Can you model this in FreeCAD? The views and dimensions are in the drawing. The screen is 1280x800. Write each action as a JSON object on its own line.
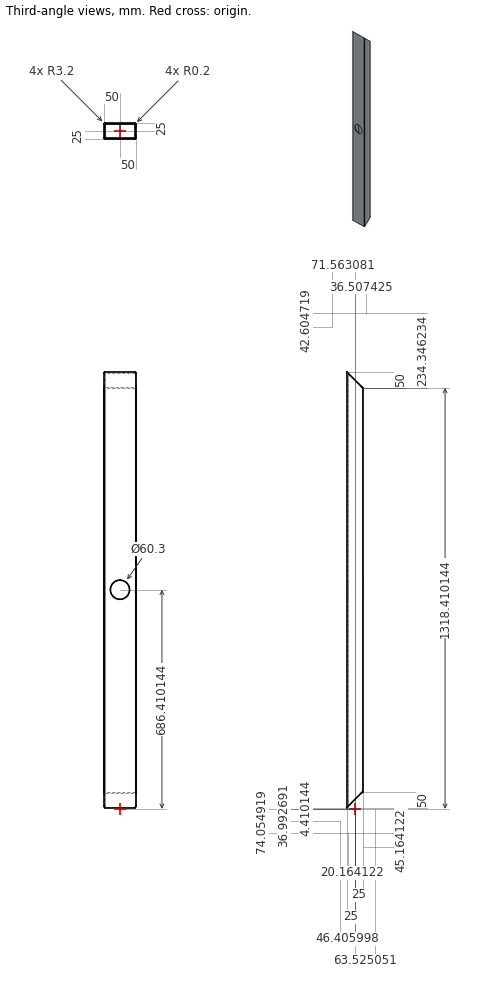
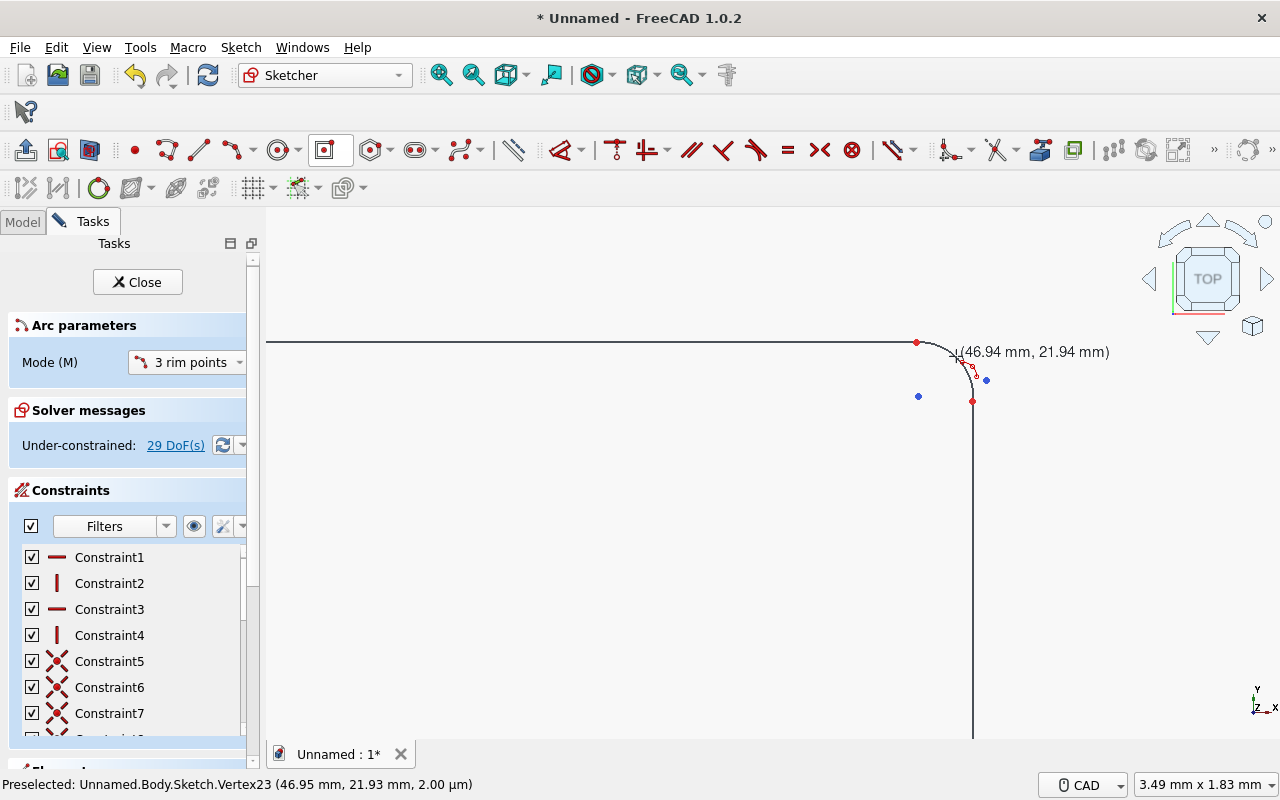
{"action": "scroll", "coordinate": [704, 473], "scroll_direction": "down", "scroll_amount": 15}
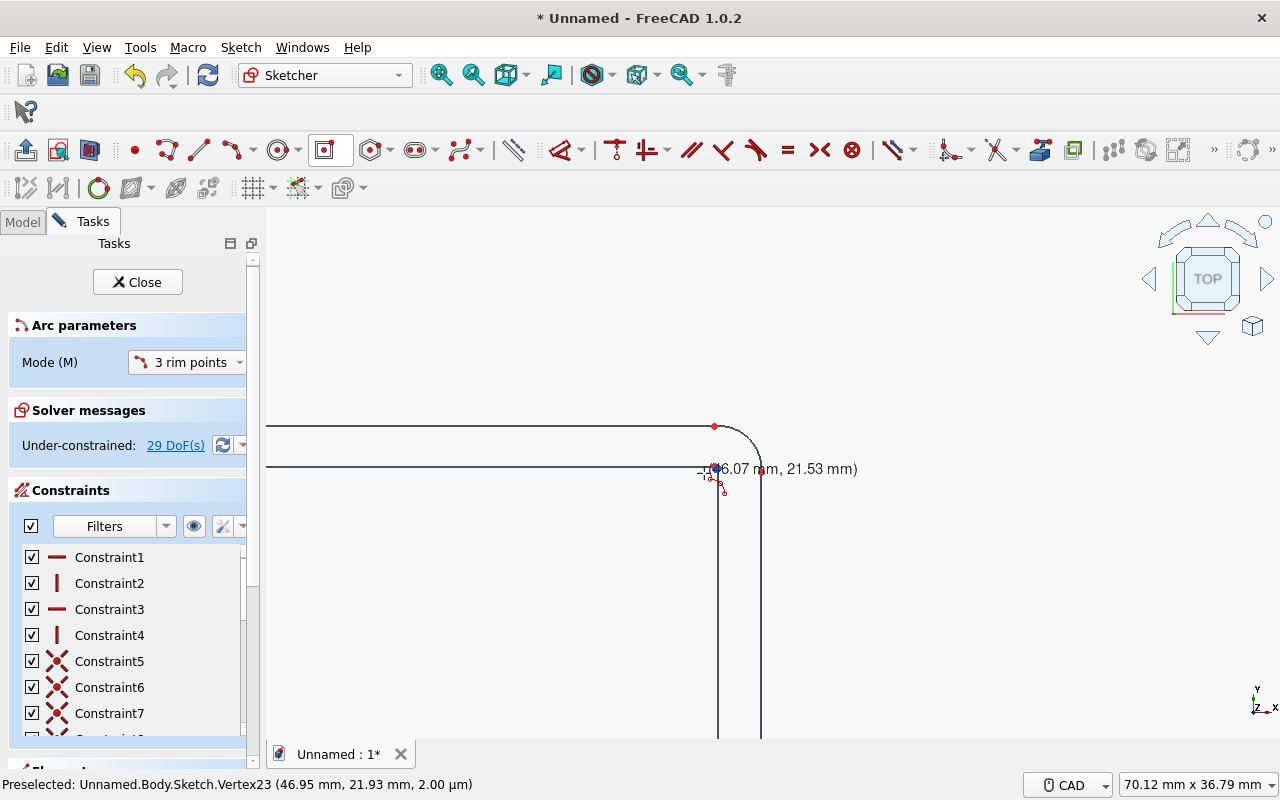
{"action": "scroll", "coordinate": [1092, 291], "scroll_direction": "down", "scroll_amount": 5}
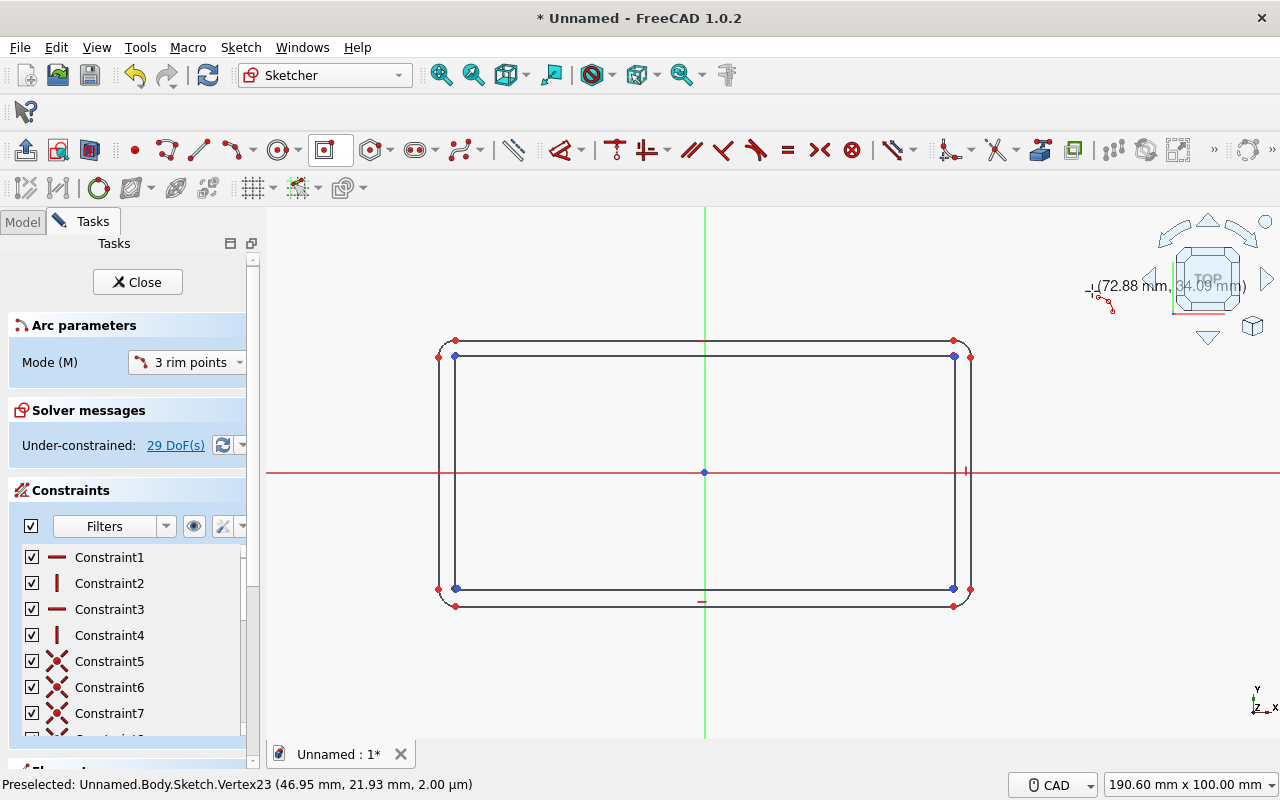
{"action": "scroll", "coordinate": [955, 589], "scroll_direction": "up", "scroll_amount": 14}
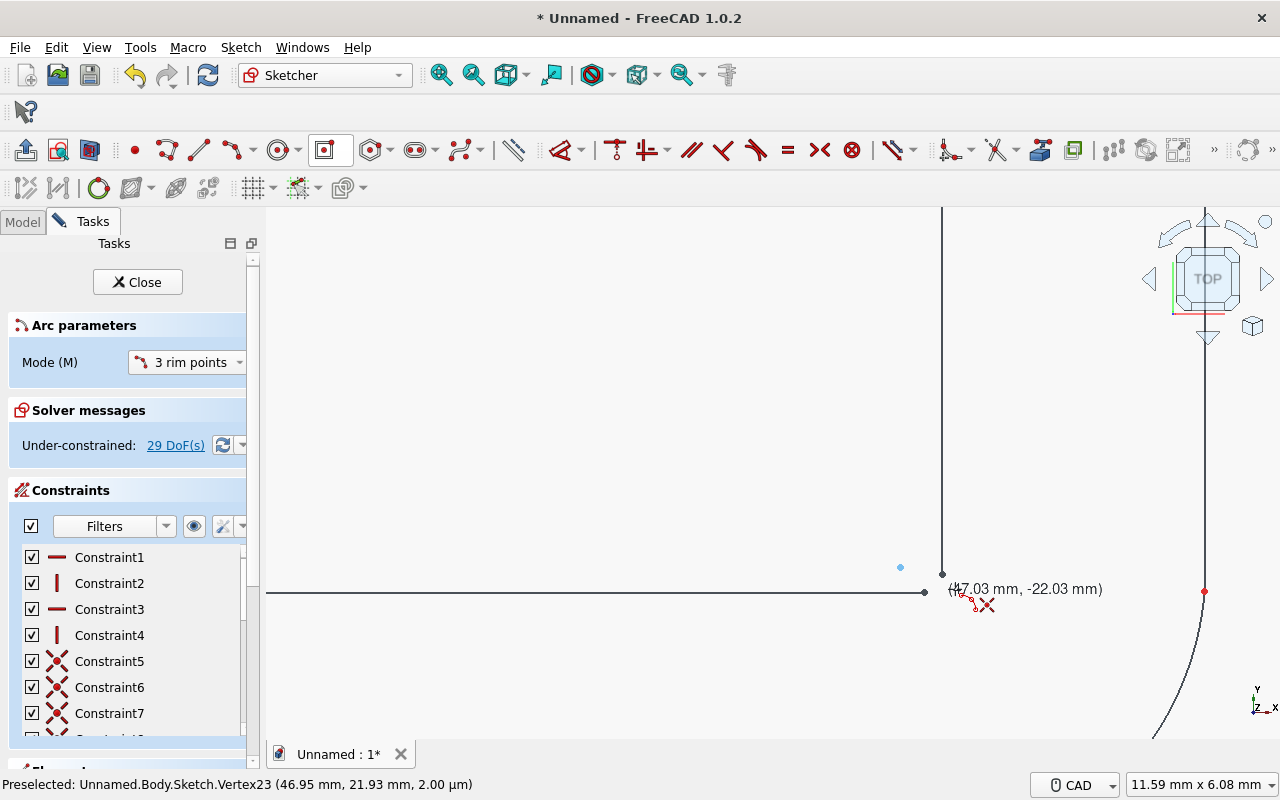
{"action": "left_click", "coordinate": [942, 575]}
{"action": "left_click", "coordinate": [925, 593]}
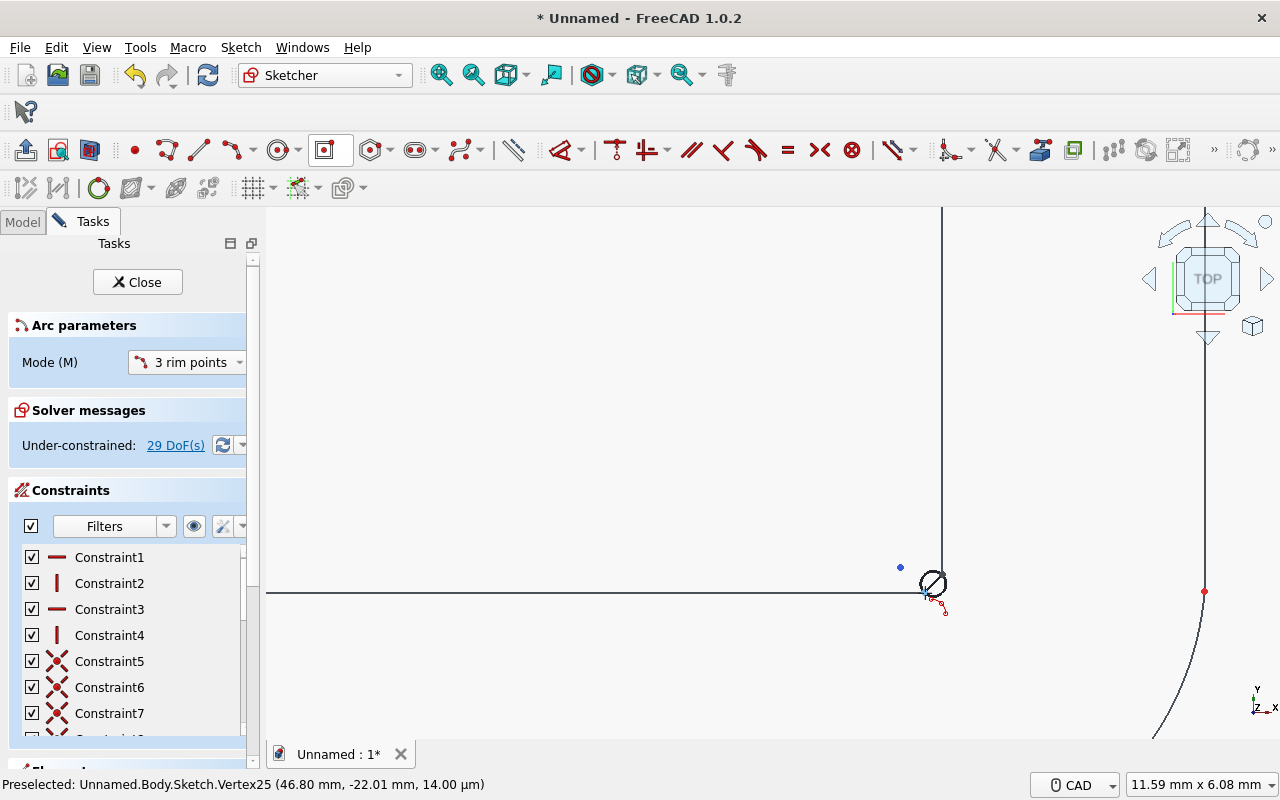
{"action": "scroll", "coordinate": [937, 587], "scroll_direction": "up", "scroll_amount": 6}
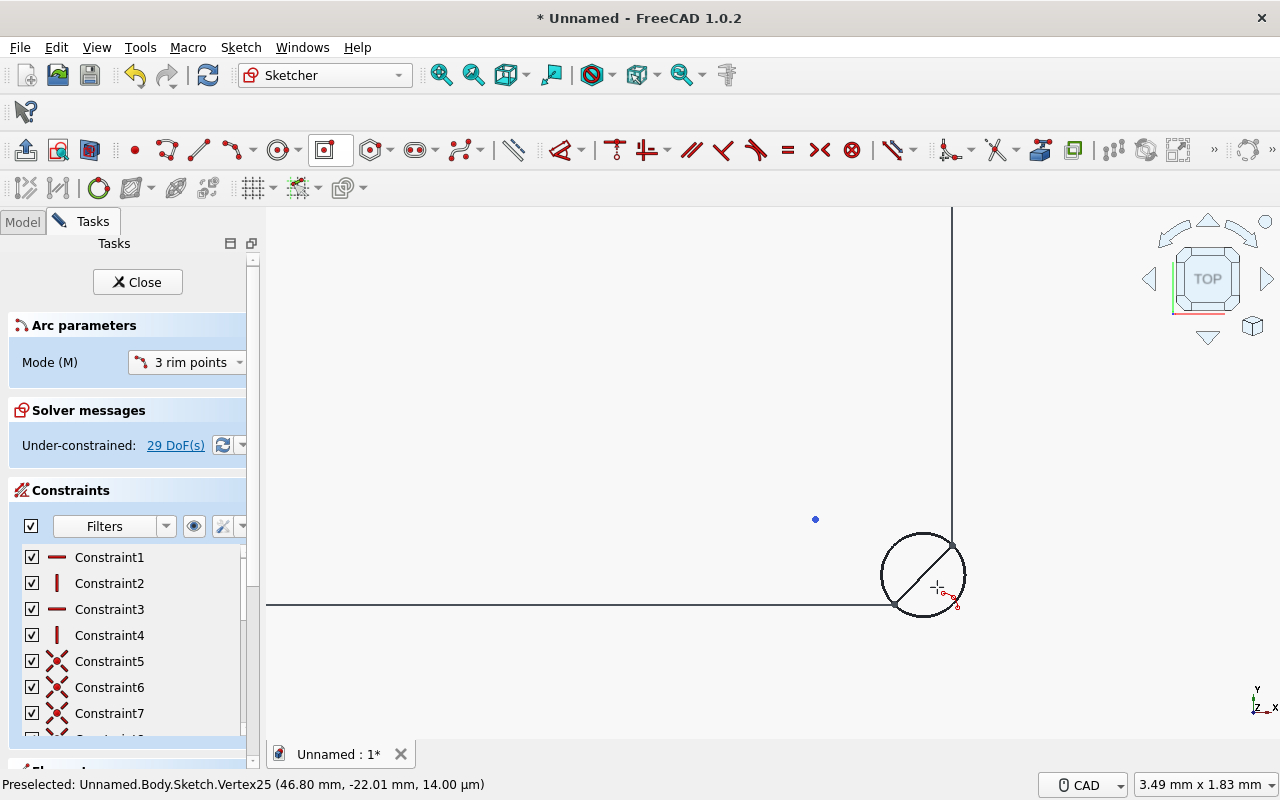
{"action": "left_click", "coordinate": [936, 585]}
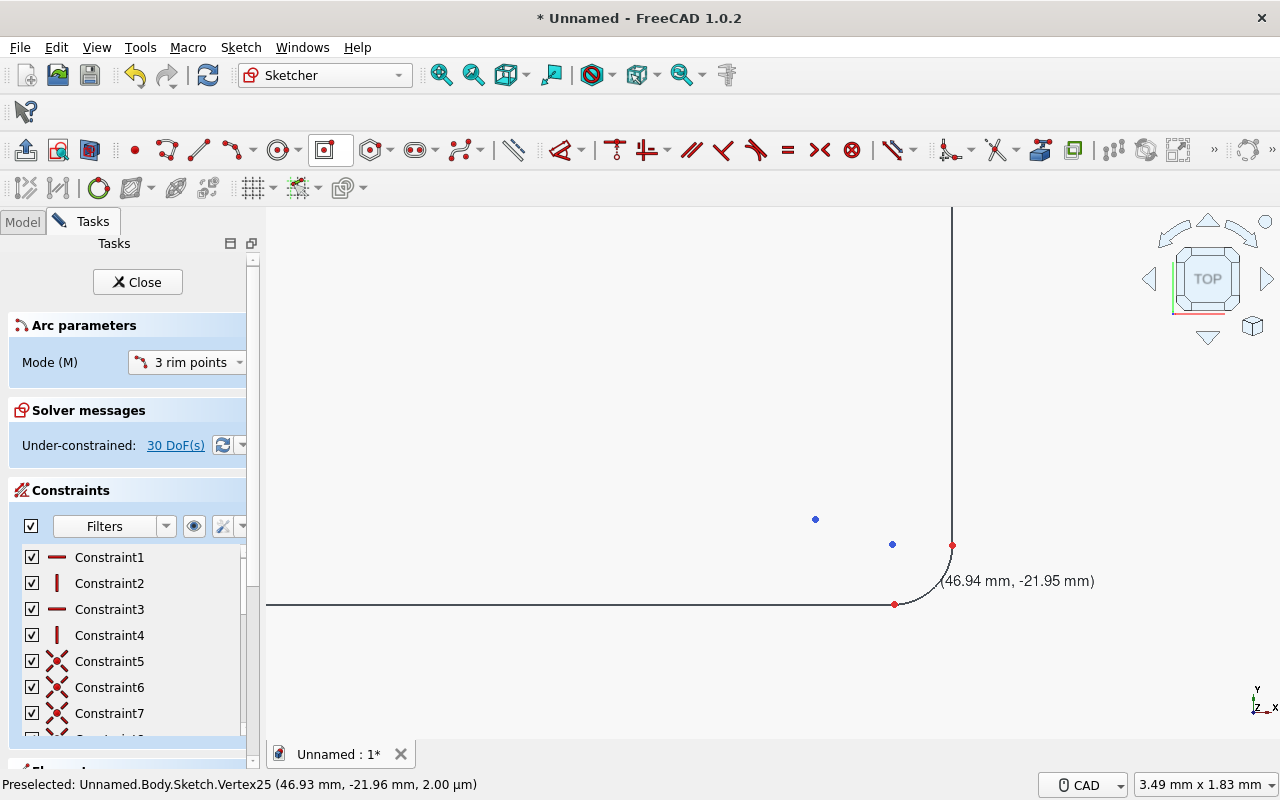
{"action": "scroll", "coordinate": [704, 473], "scroll_direction": "down", "scroll_amount": 15}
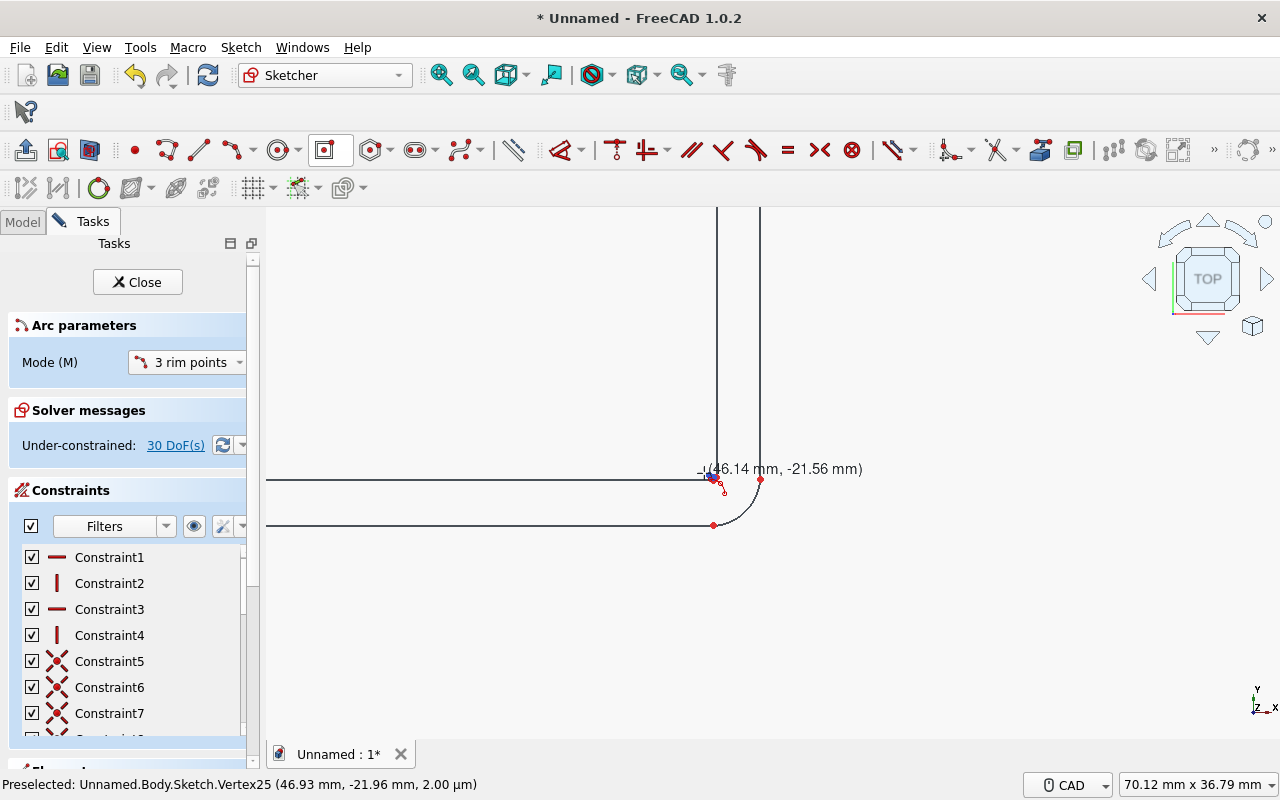
{"action": "scroll", "coordinate": [1093, 654], "scroll_direction": "down", "scroll_amount": 5}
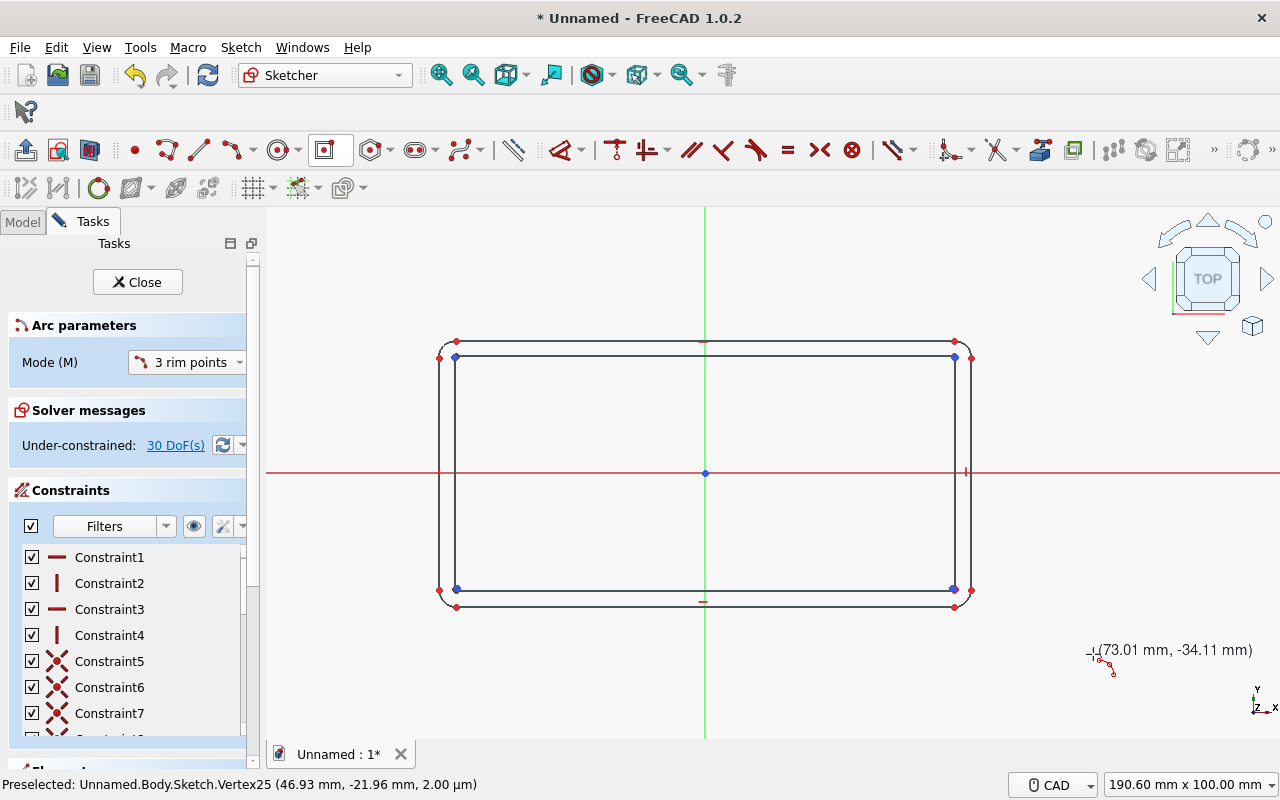
{"action": "scroll", "coordinate": [456, 590], "scroll_direction": "up", "scroll_amount": 14}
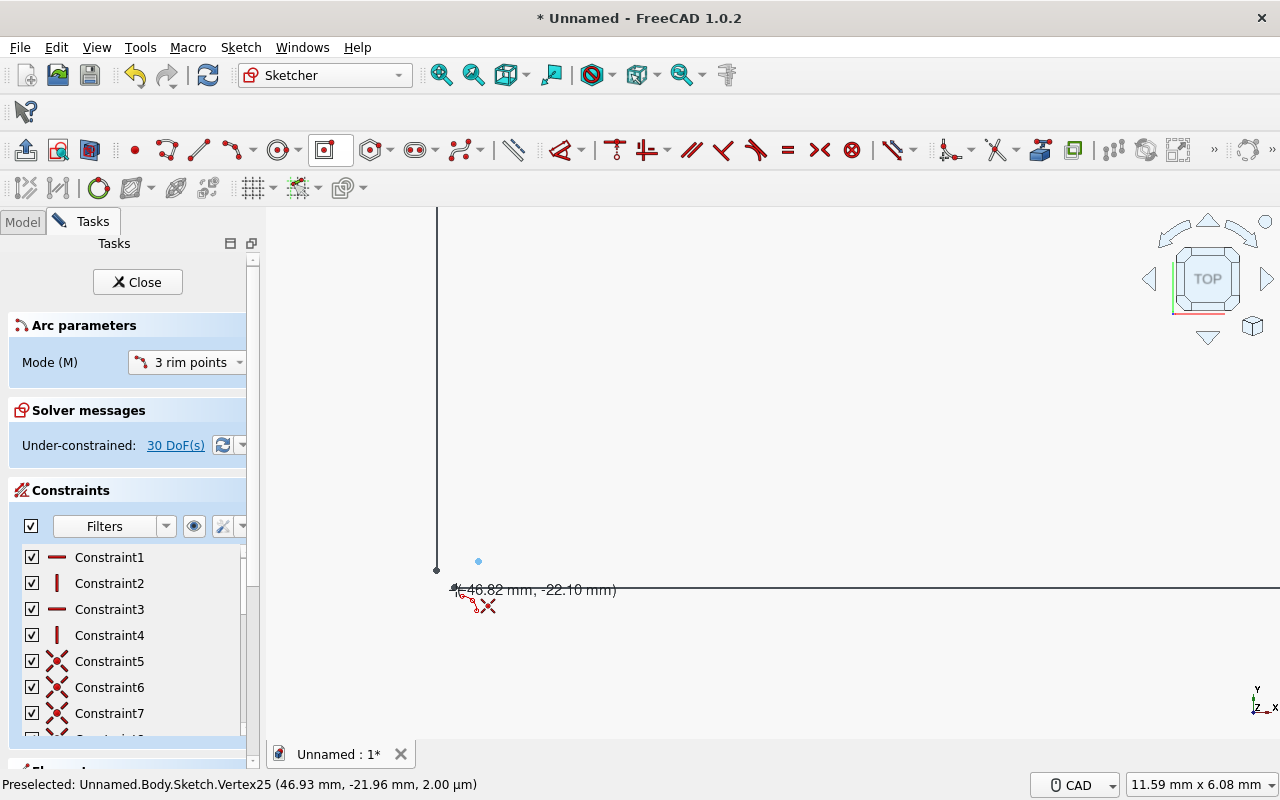
{"action": "left_click", "coordinate": [455, 588]}
{"action": "left_click", "coordinate": [437, 570]}